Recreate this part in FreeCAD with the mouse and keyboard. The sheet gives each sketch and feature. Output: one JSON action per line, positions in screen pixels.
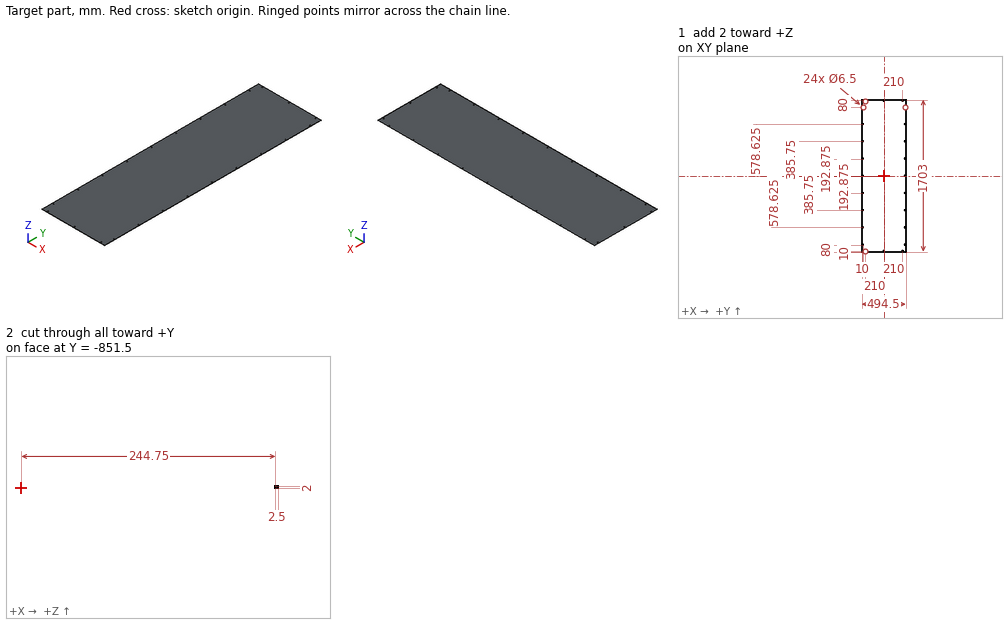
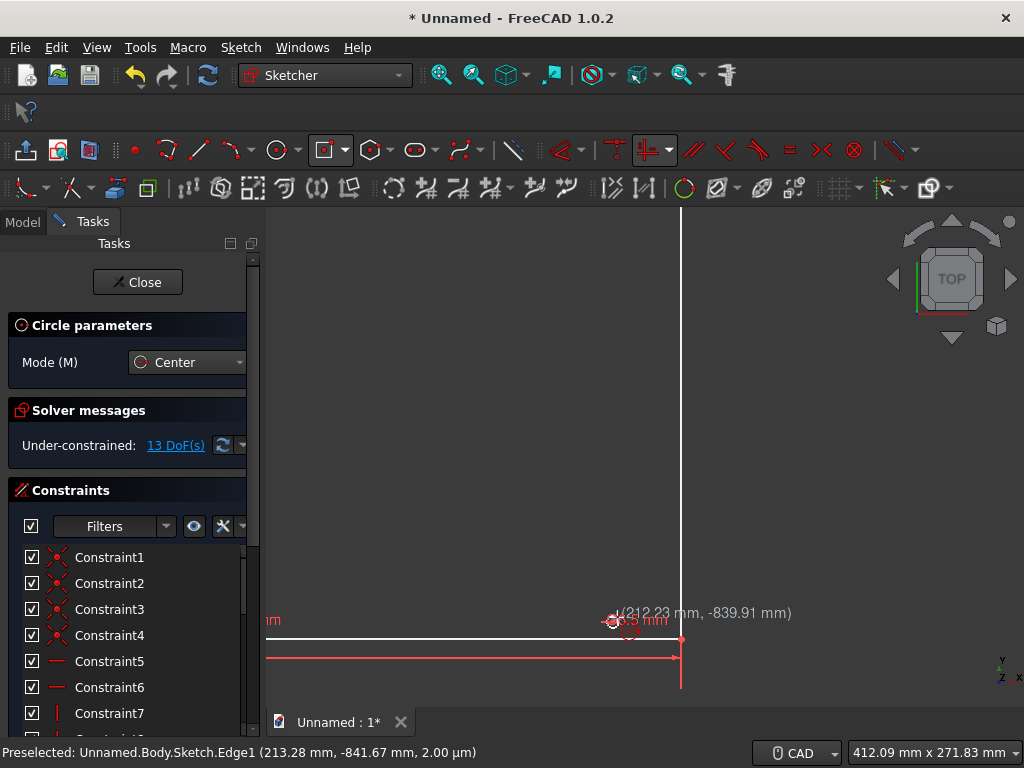
{"action": "scroll", "coordinate": [663, 492], "scroll_direction": "up", "scroll_amount": 7}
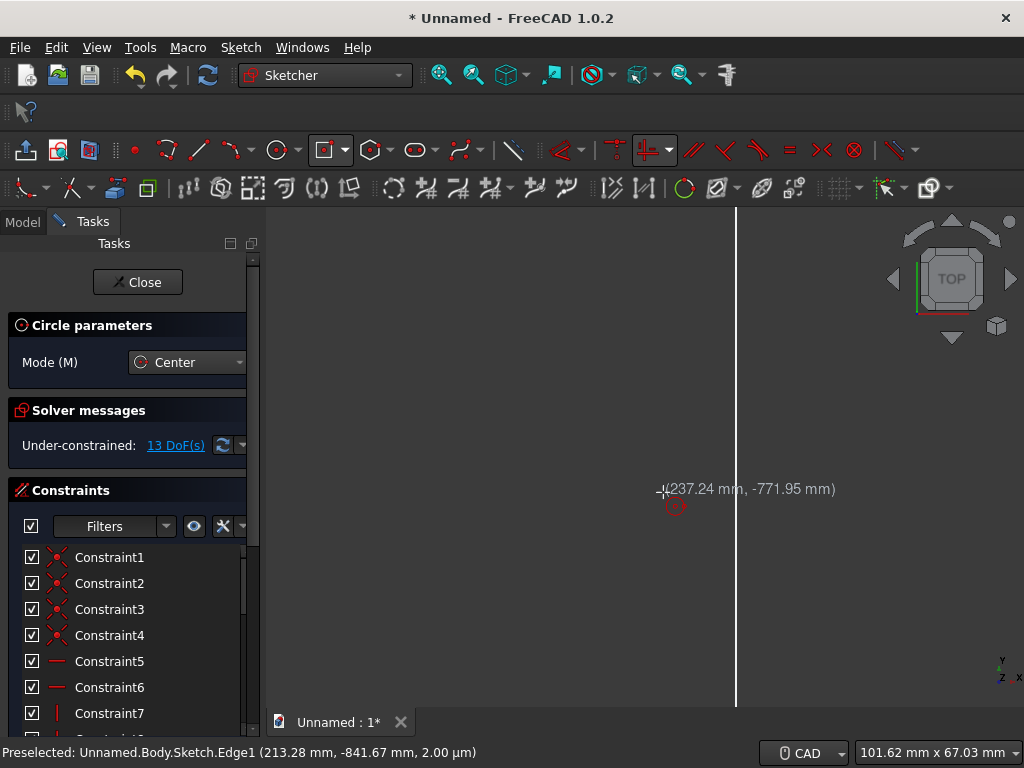
{"action": "scroll", "coordinate": [624, 618], "scroll_direction": "down", "scroll_amount": 18}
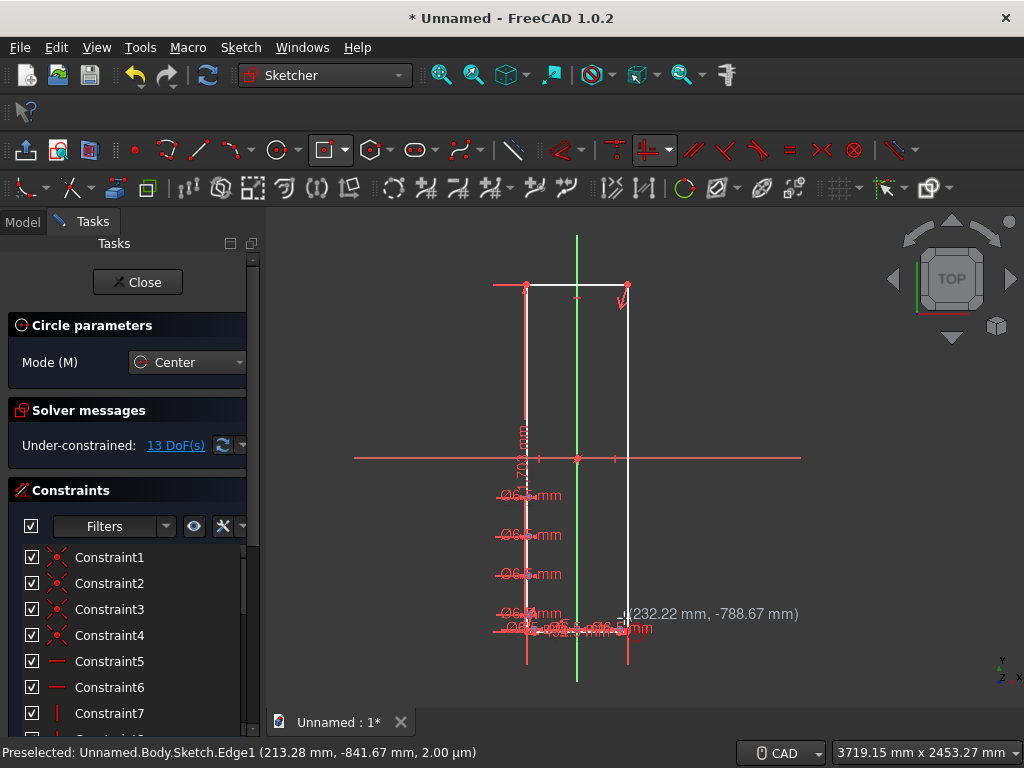
{"action": "scroll", "coordinate": [625, 615], "scroll_direction": "up", "scroll_amount": 11}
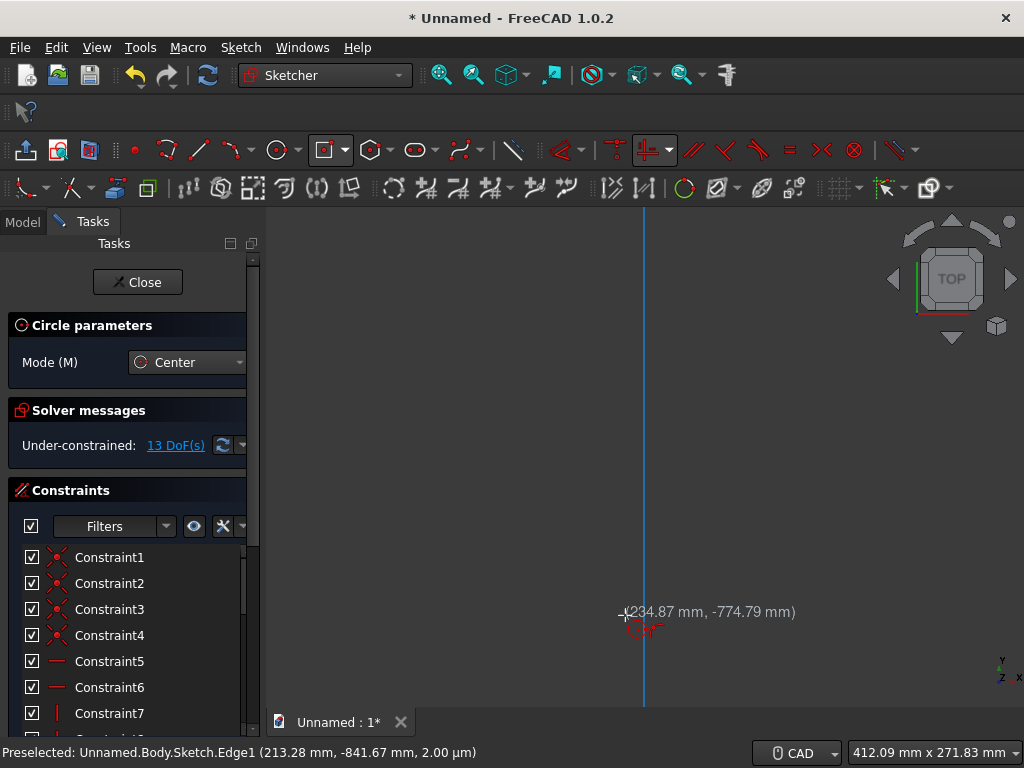
{"action": "left_click", "coordinate": [626, 611]}
{"action": "mouse_move", "coordinate": [630, 607]}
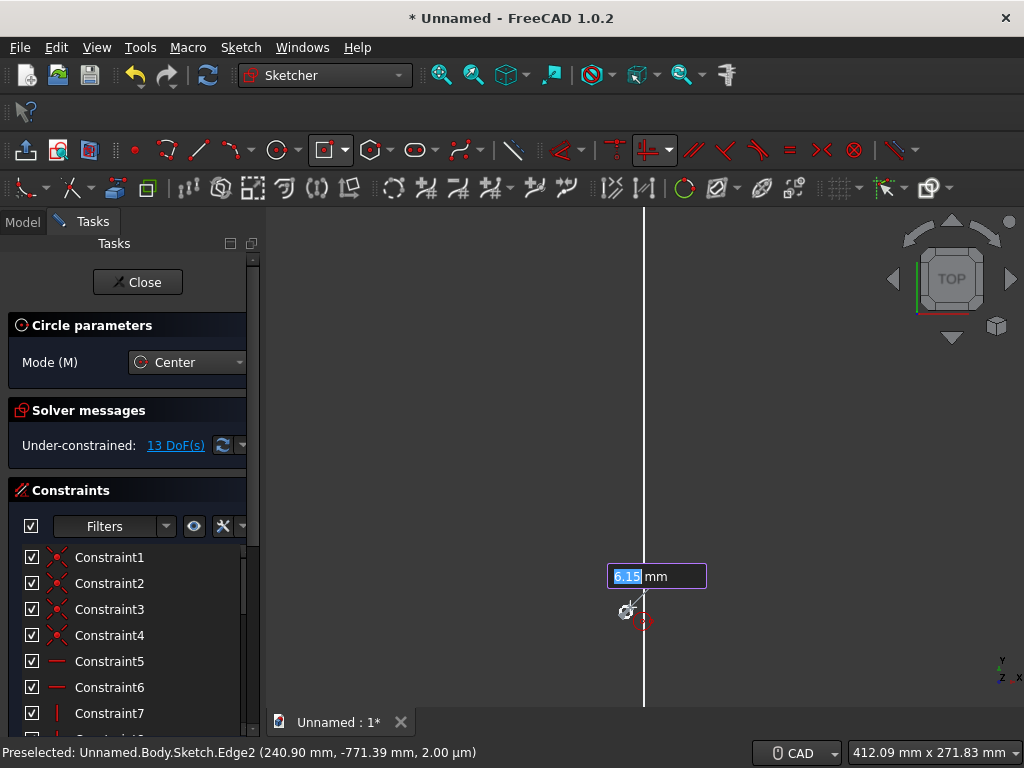
{"action": "type", "text": "6.5"}
{"action": "key", "text": "Return"}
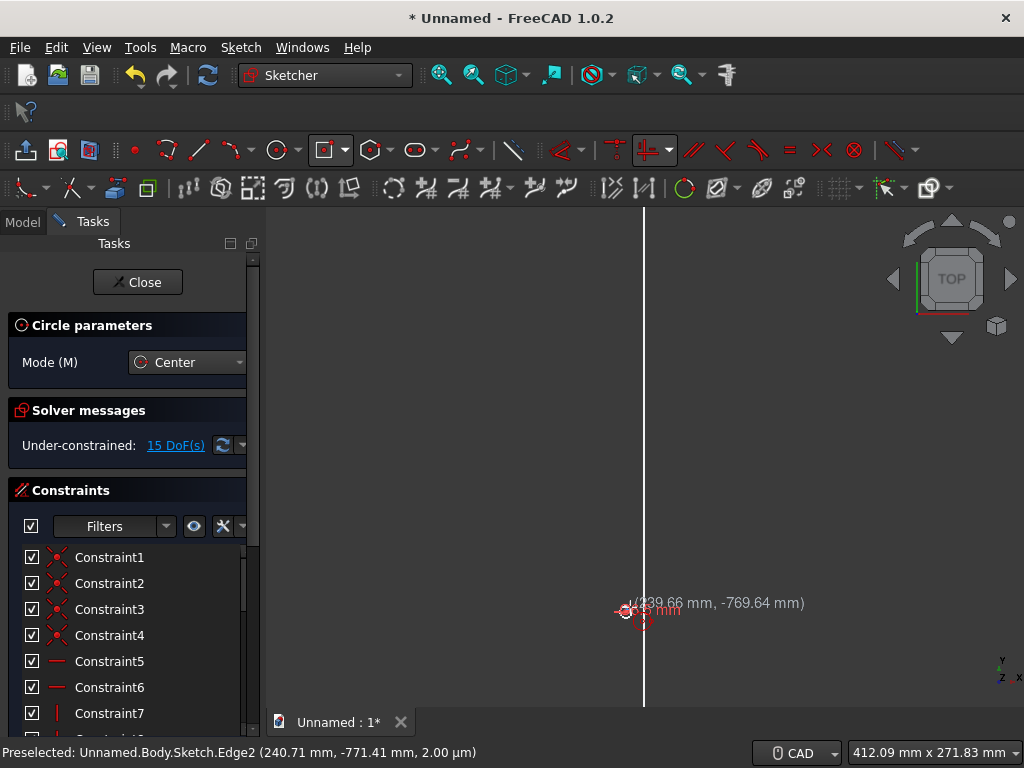
{"action": "scroll", "coordinate": [626, 257], "scroll_direction": "up", "scroll_amount": 7}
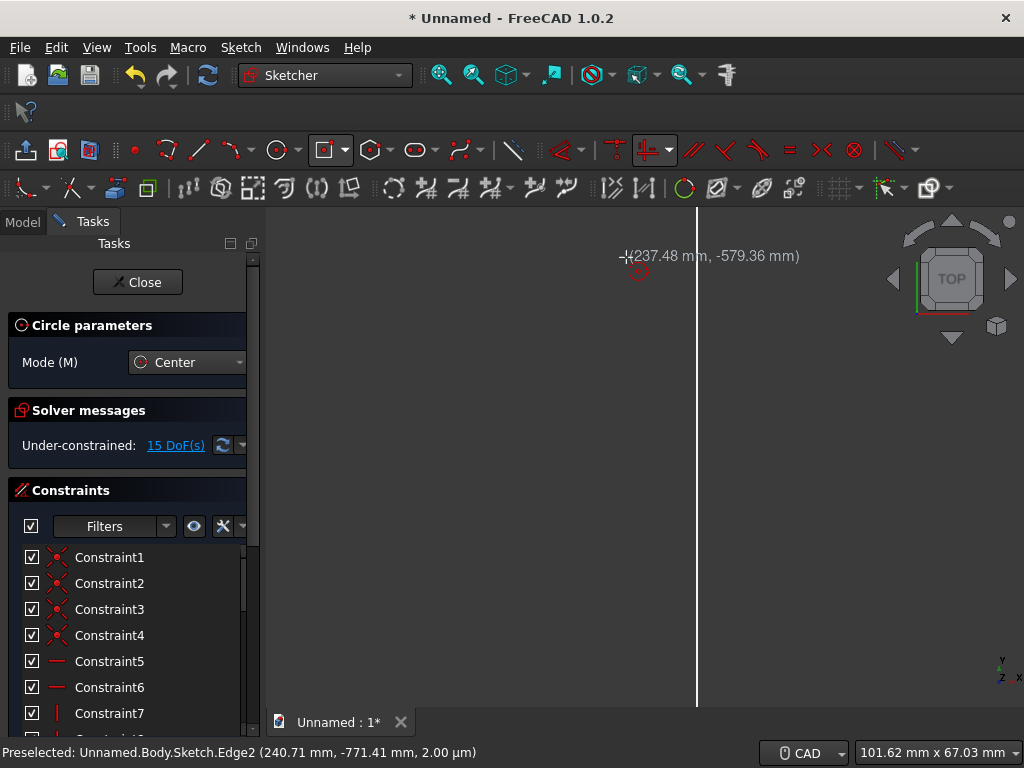
{"action": "scroll", "coordinate": [625, 584], "scroll_direction": "down", "scroll_amount": 18}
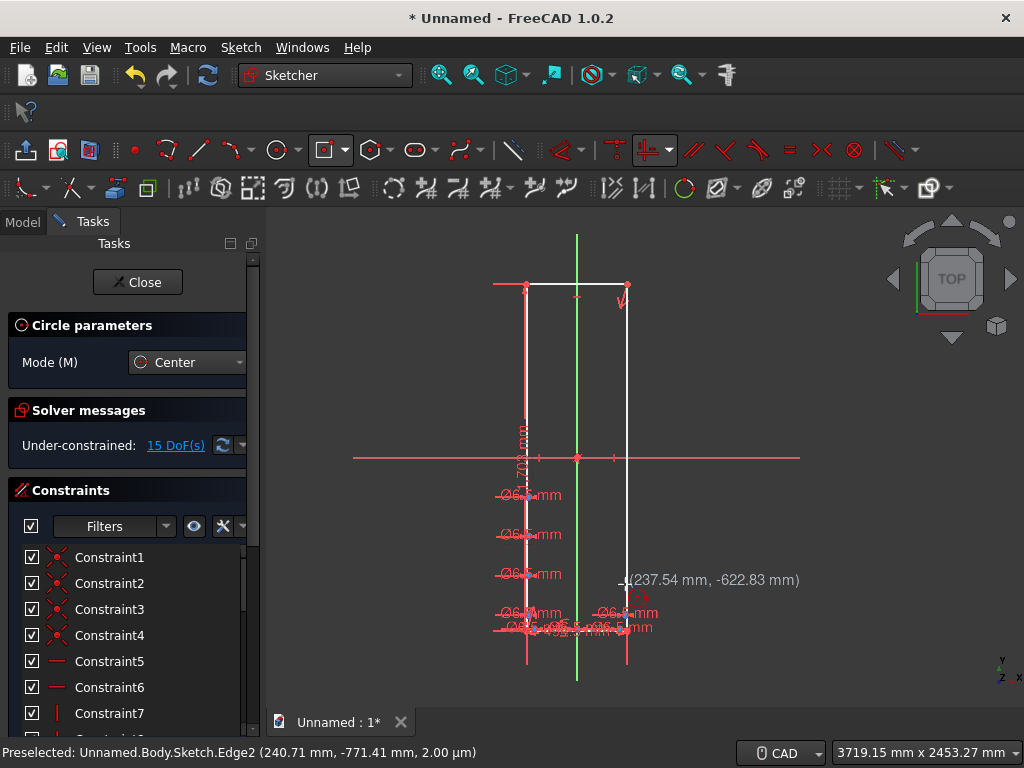
{"action": "scroll", "coordinate": [625, 576], "scroll_direction": "up", "scroll_amount": 11}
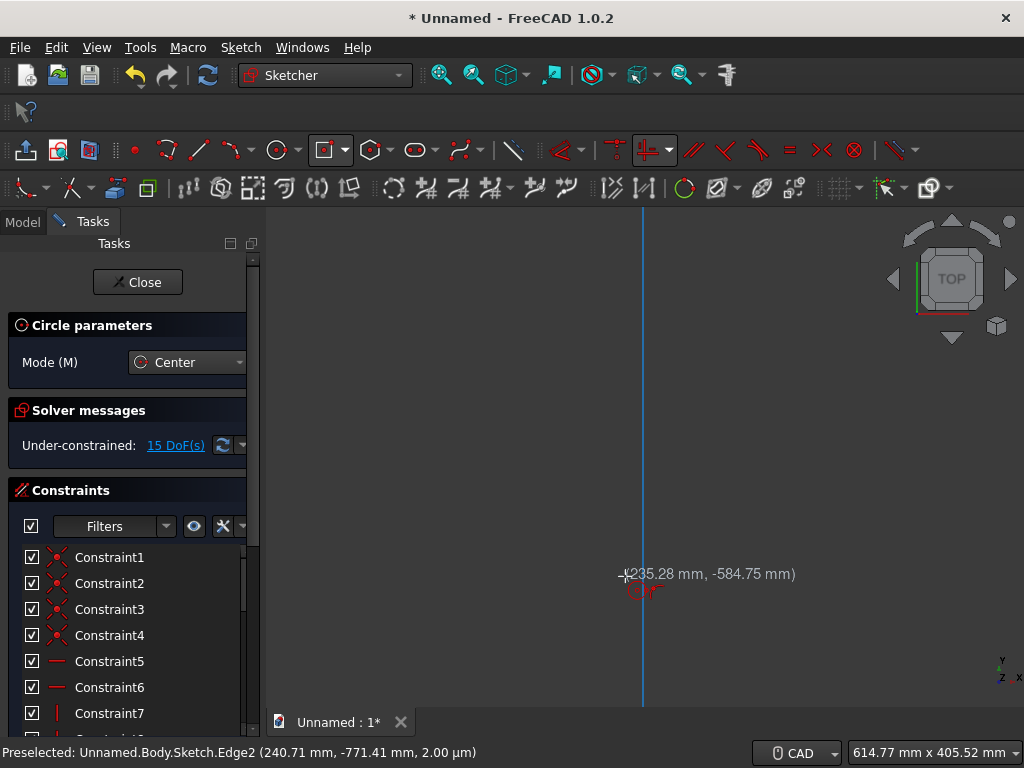
{"action": "left_click", "coordinate": [625, 568]}
{"action": "mouse_move", "coordinate": [629, 564]}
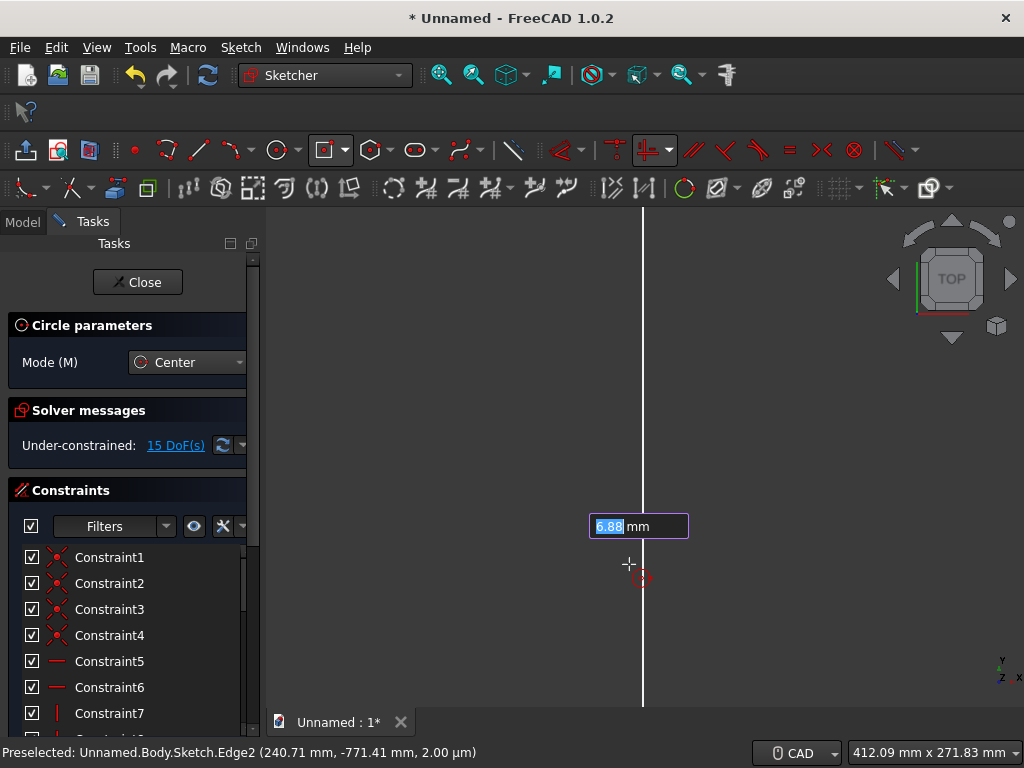
{"action": "type", "text": "6.5"}
{"action": "key", "text": "Return"}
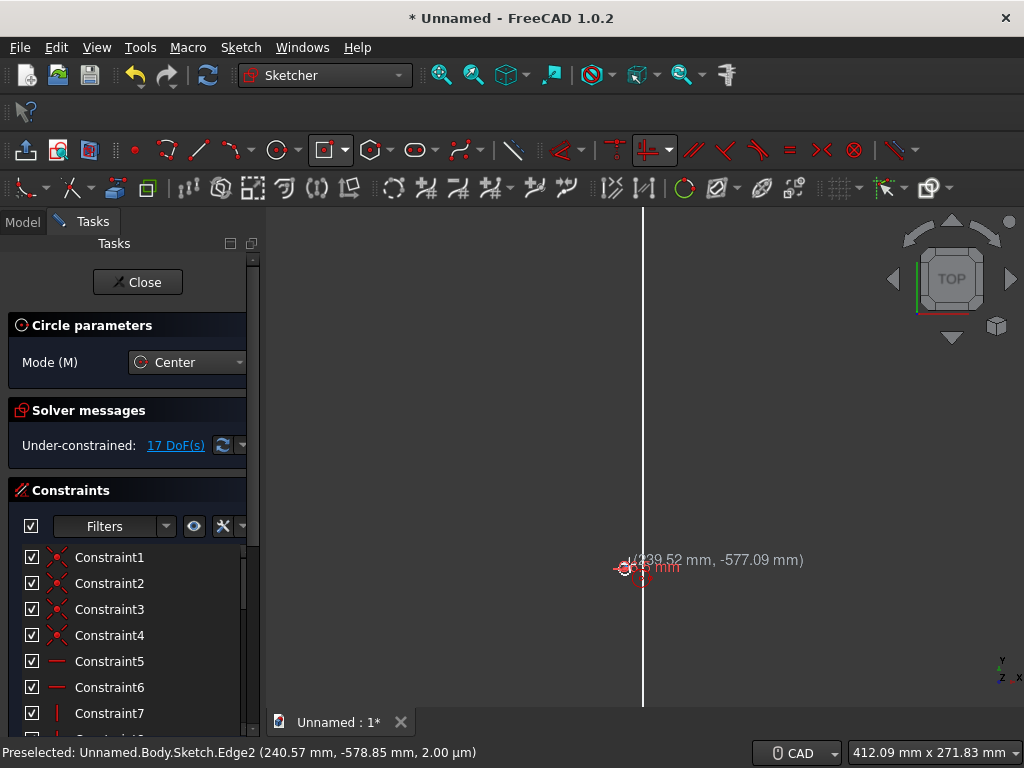
{"action": "scroll", "coordinate": [615, 552], "scroll_direction": "down", "scroll_amount": 12}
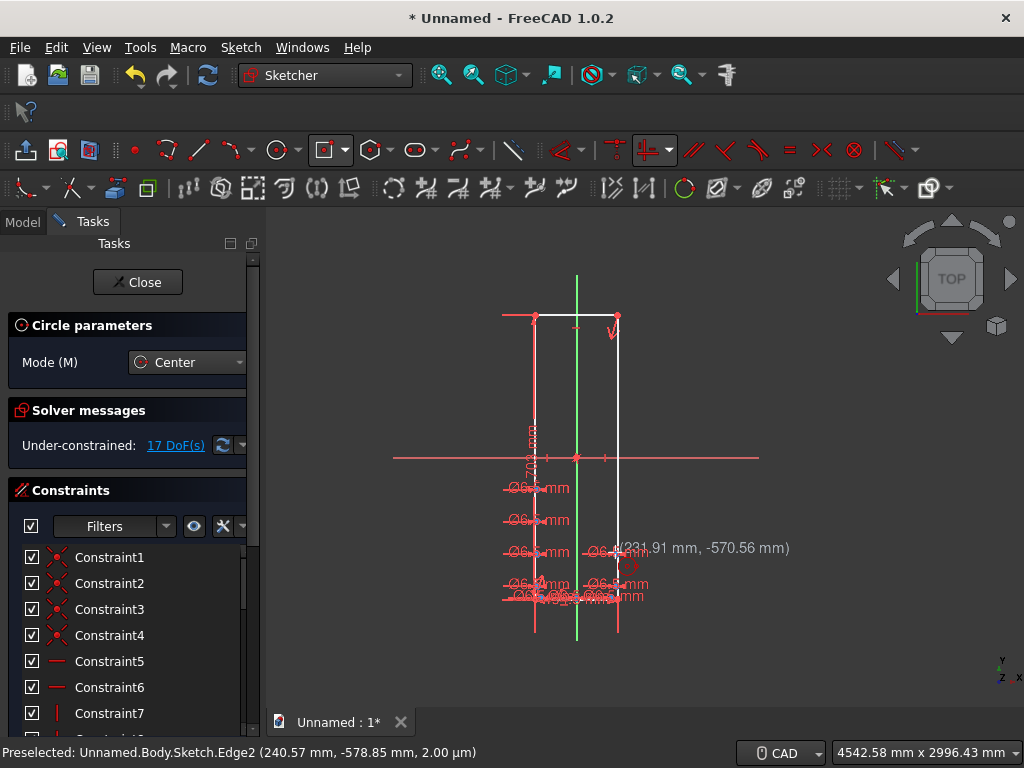
{"action": "scroll", "coordinate": [616, 522], "scroll_direction": "up", "scroll_amount": 19}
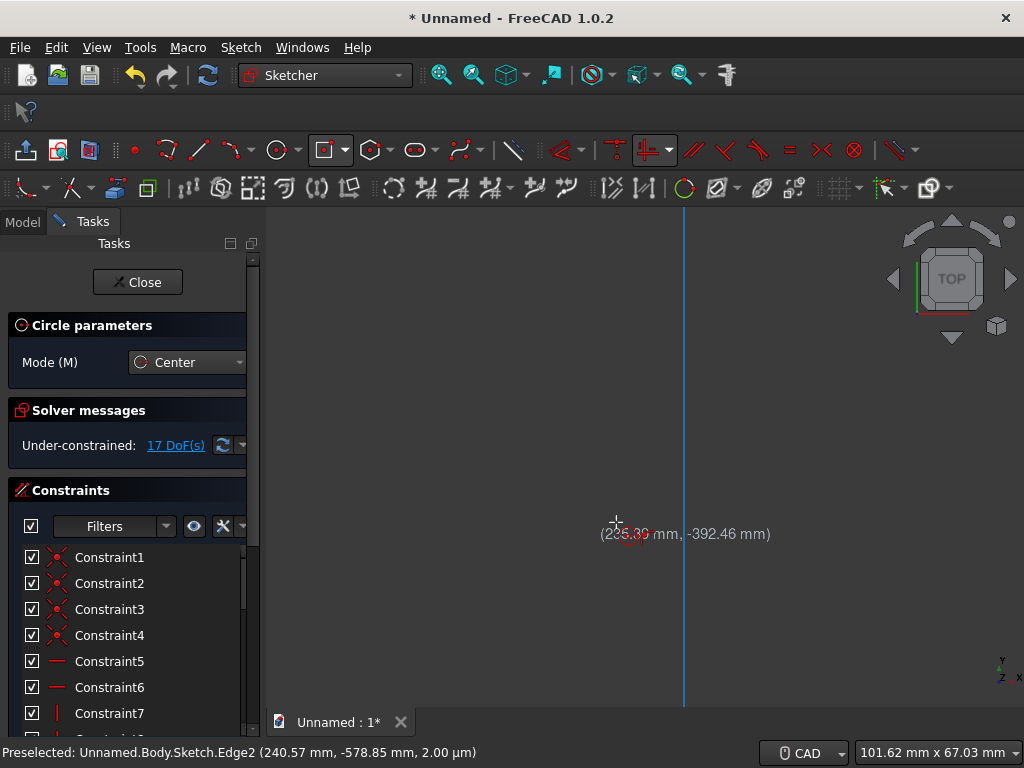
{"action": "scroll", "coordinate": [625, 537], "scroll_direction": "down", "scroll_amount": 18}